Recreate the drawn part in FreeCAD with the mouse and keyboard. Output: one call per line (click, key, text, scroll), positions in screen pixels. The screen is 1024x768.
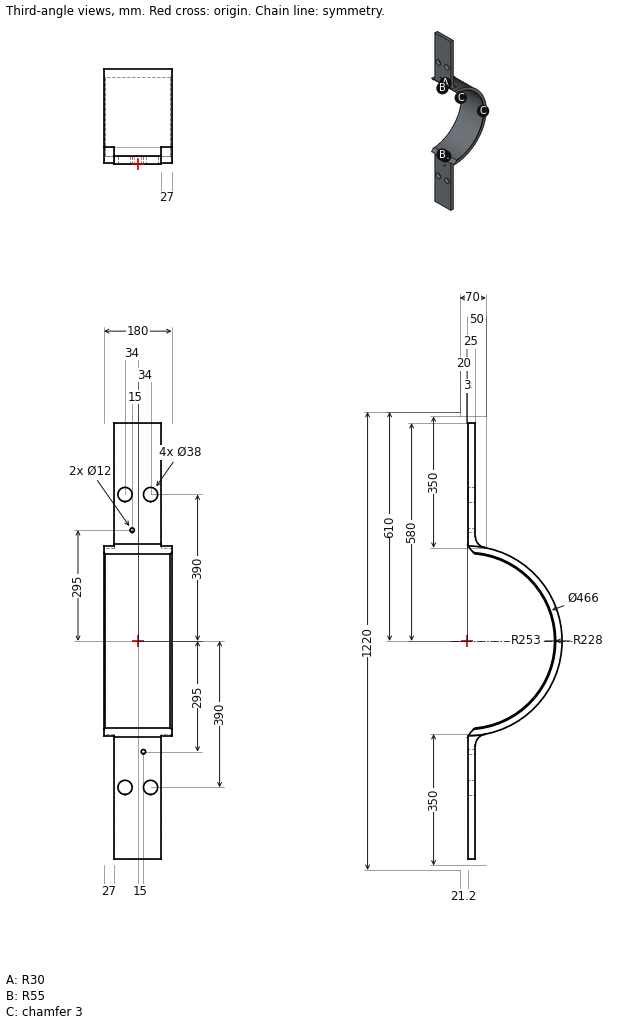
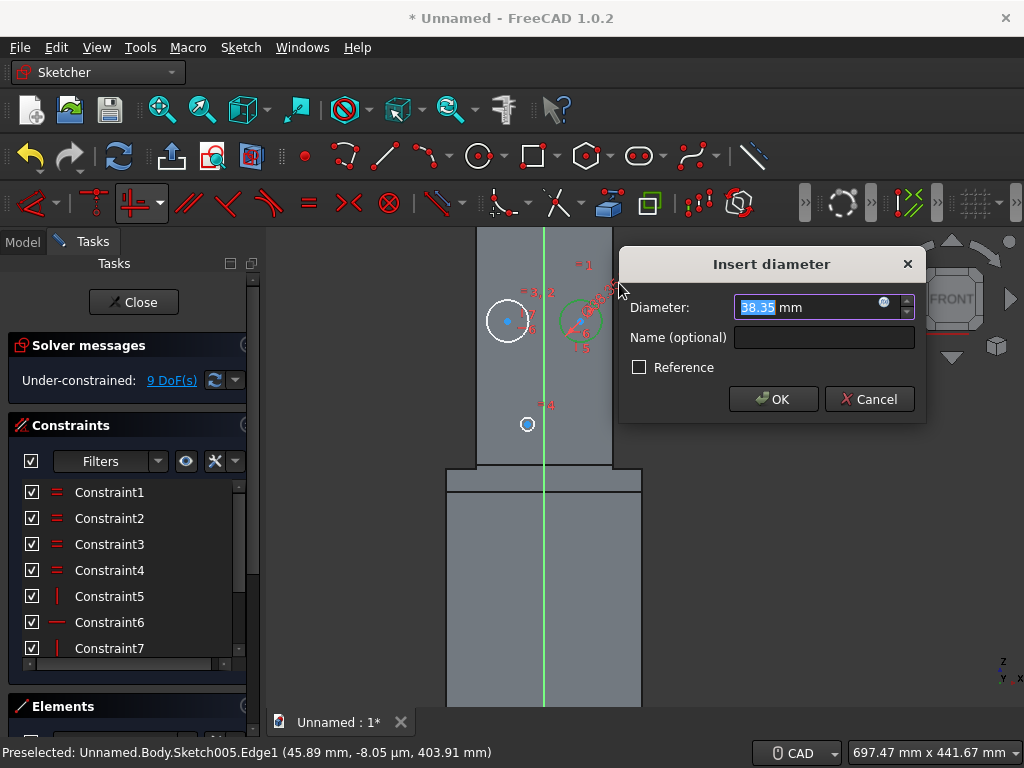
text(38)
key(Return)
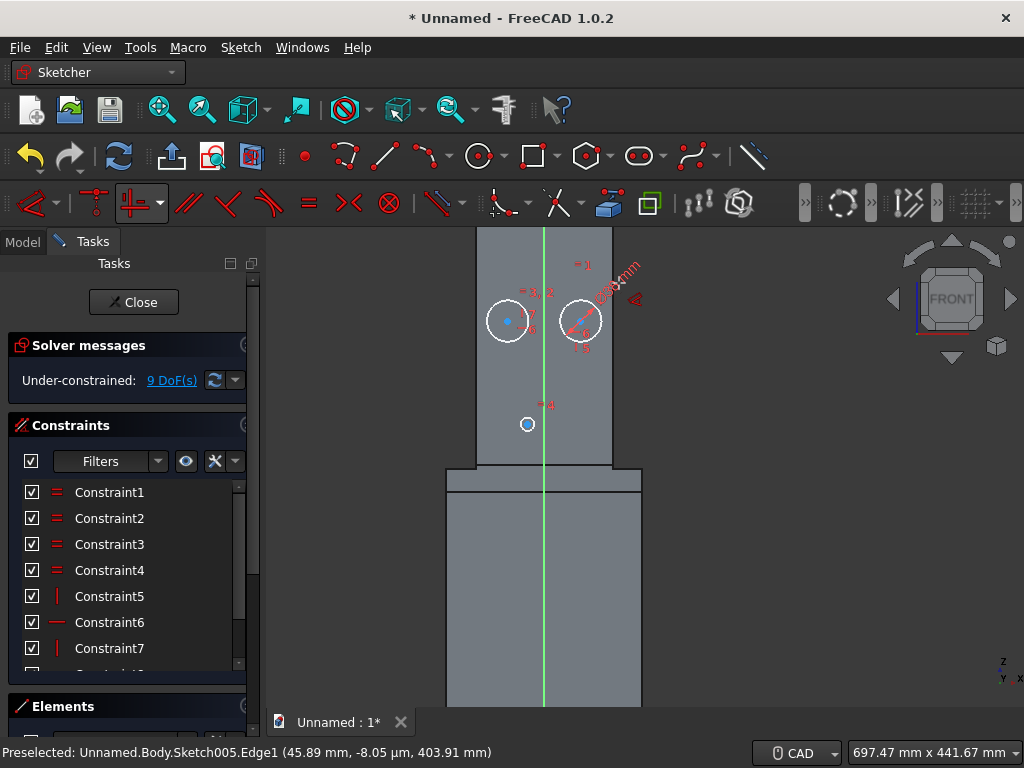
scroll(532, 419, up, 6)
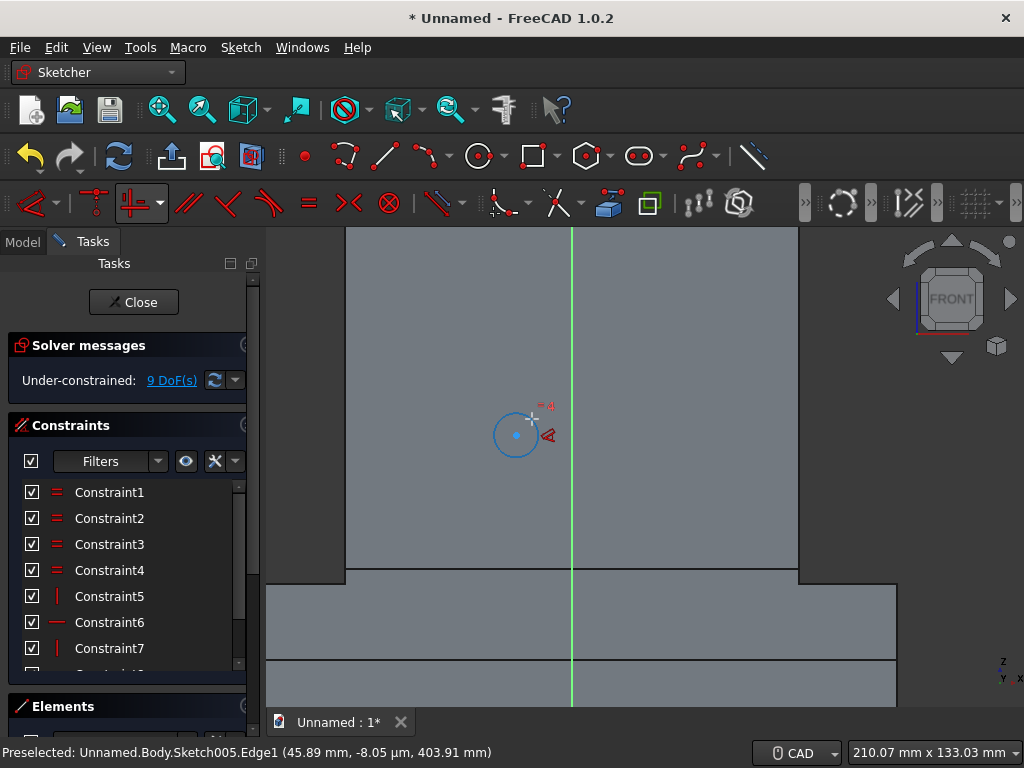
click(532, 420)
click(555, 398)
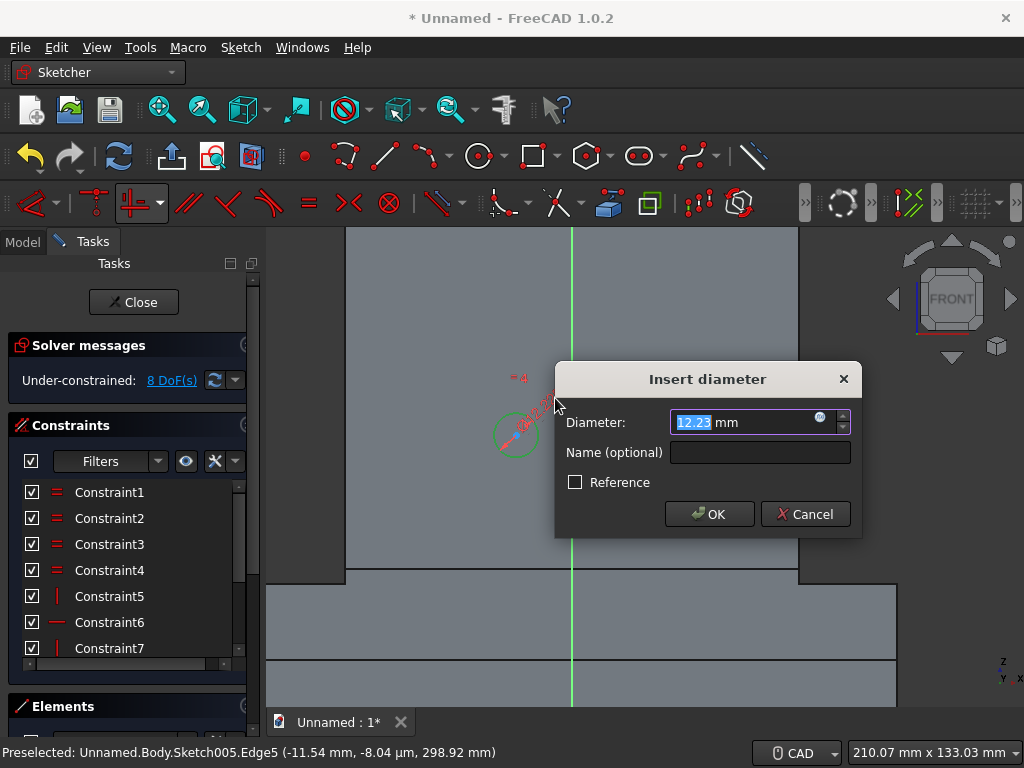
text(12)
key(Return)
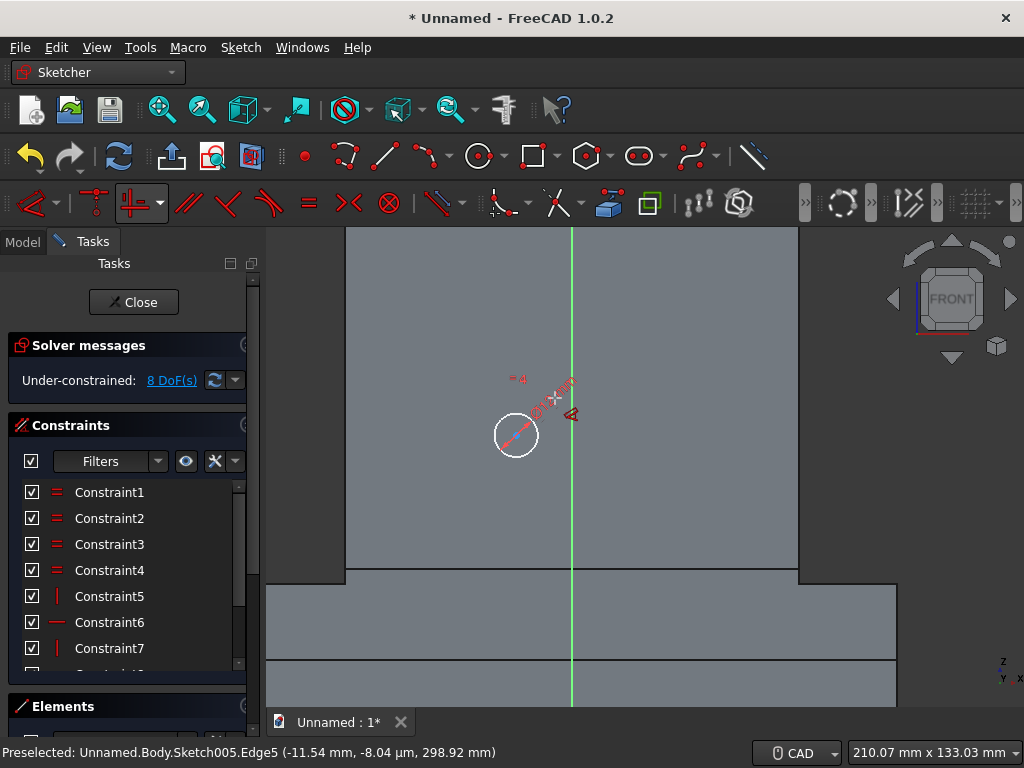
scroll(577, 339, down, 11)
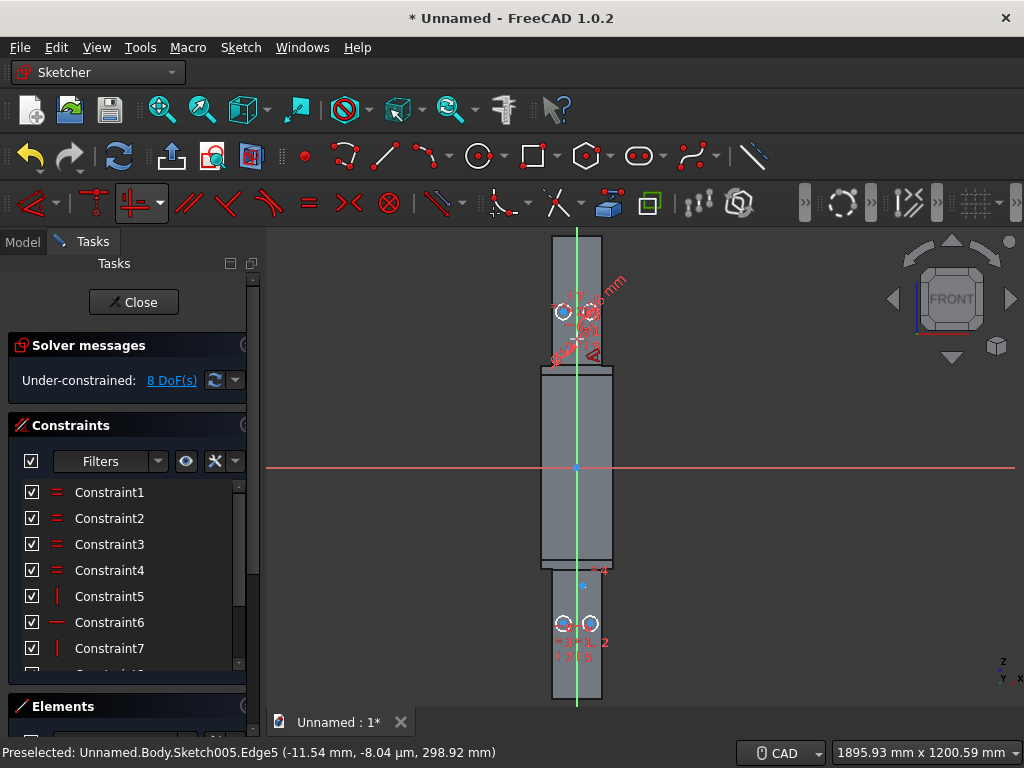
scroll(590, 312, up, 6)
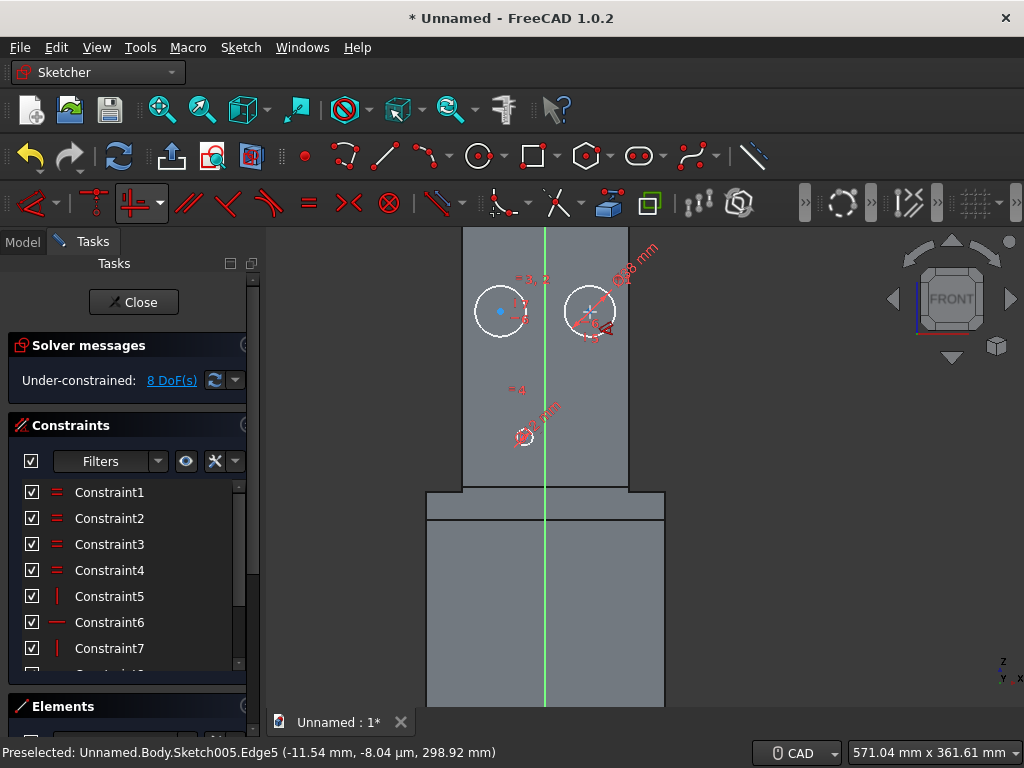
click(590, 311)
click(568, 277)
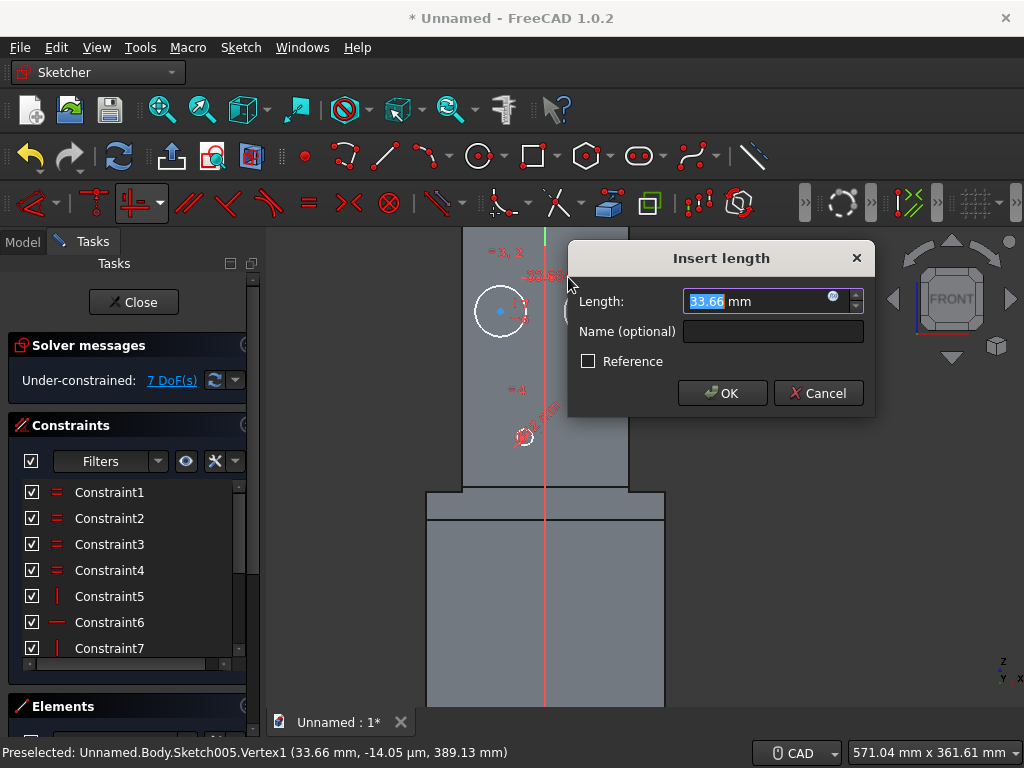
text(34)
key(Return)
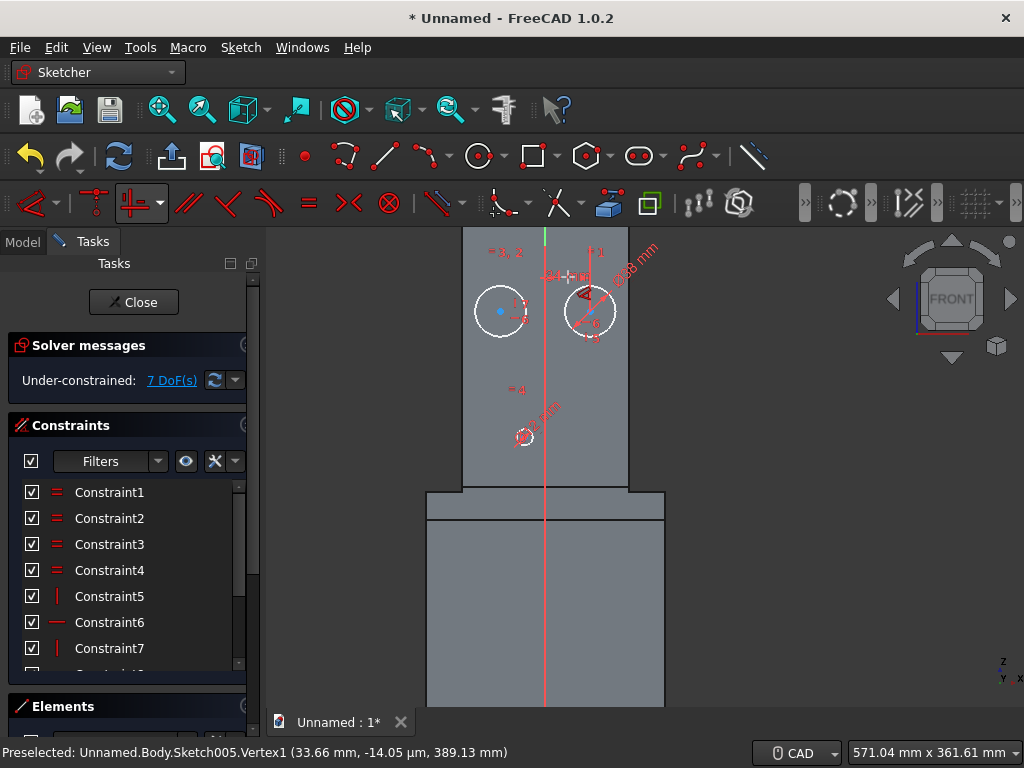
click(501, 311)
click(523, 277)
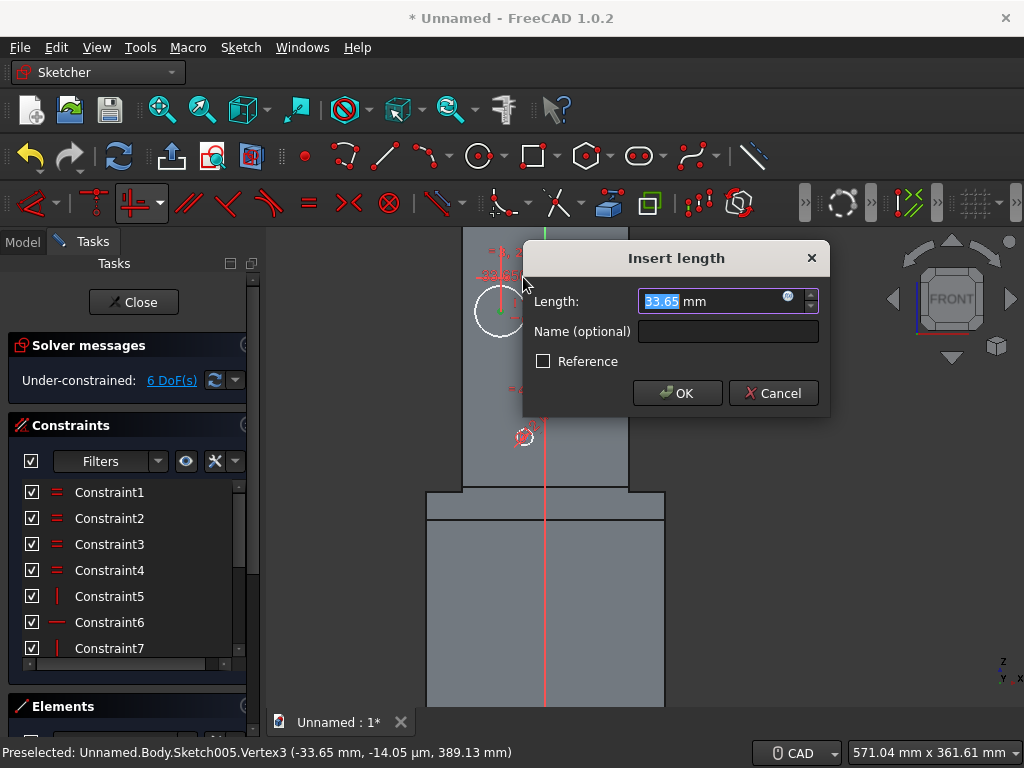
text(34)
key(Return)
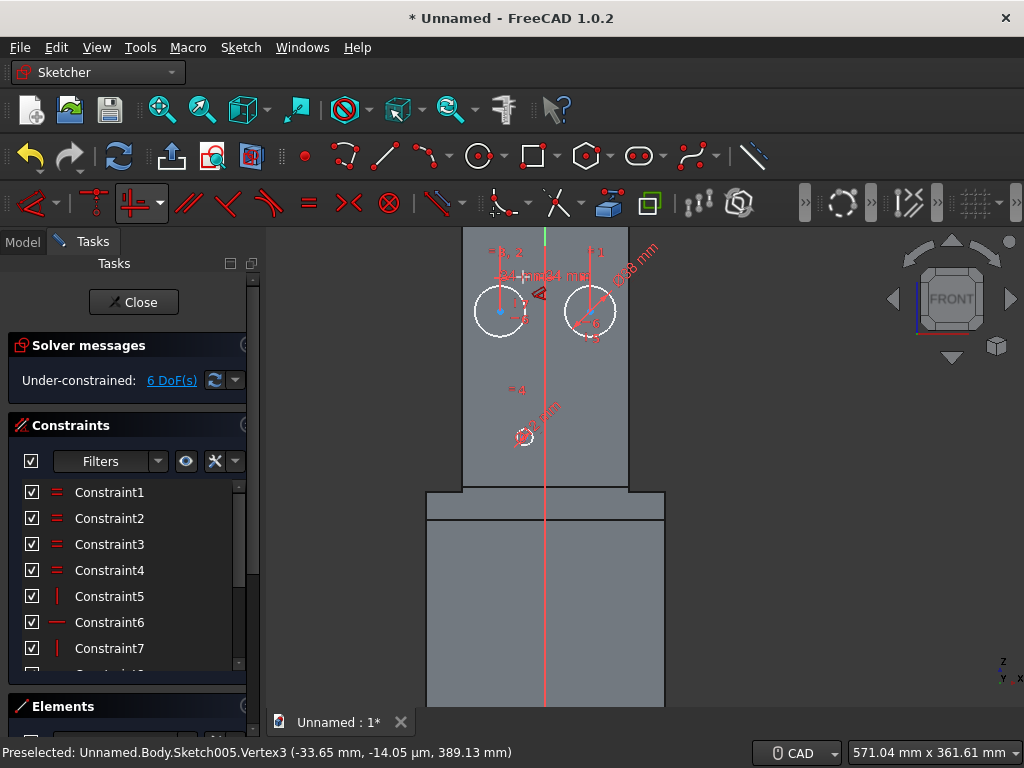
scroll(525, 437, up, 4)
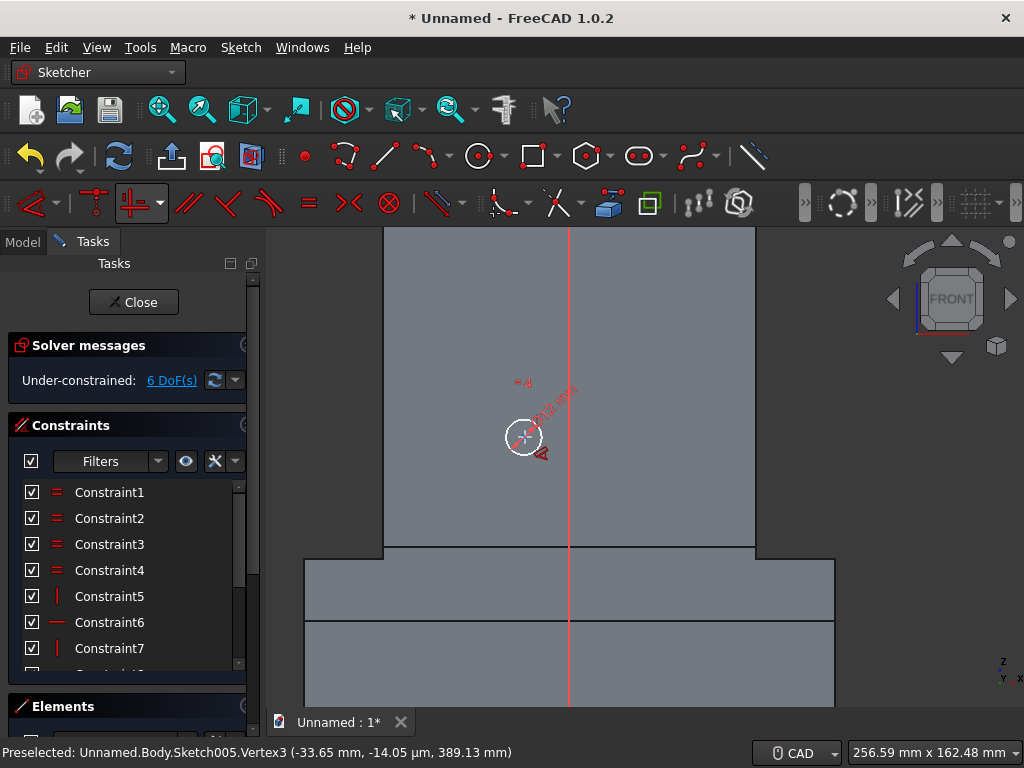
click(524, 437)
click(547, 379)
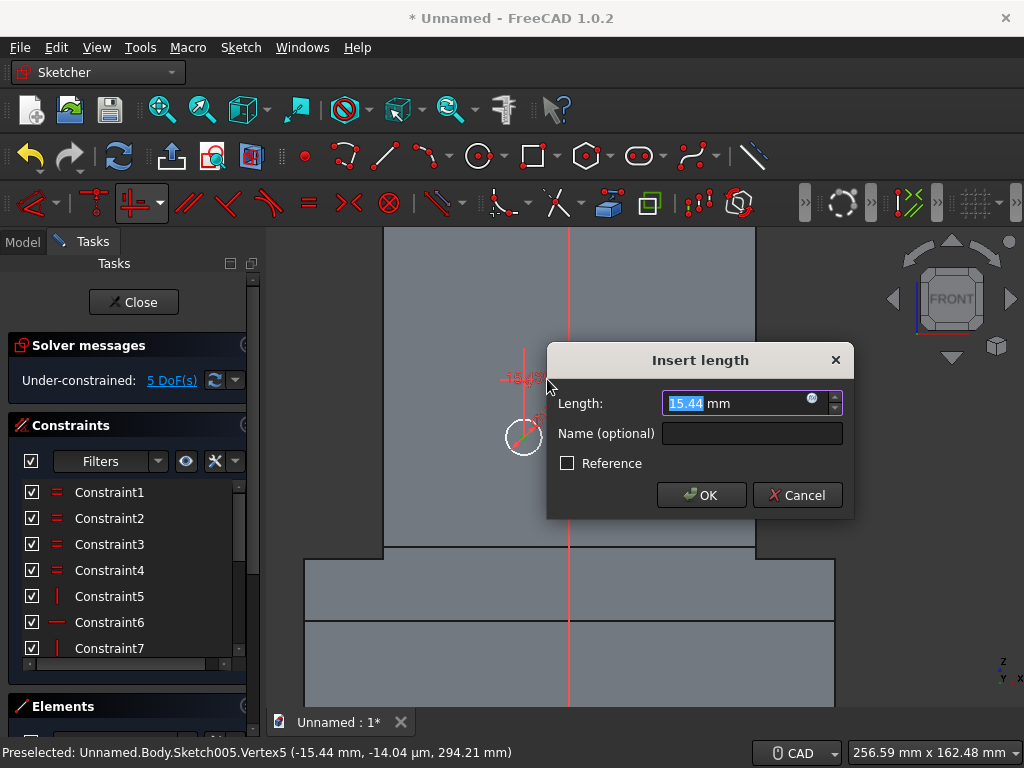
text(15)
key(Return)